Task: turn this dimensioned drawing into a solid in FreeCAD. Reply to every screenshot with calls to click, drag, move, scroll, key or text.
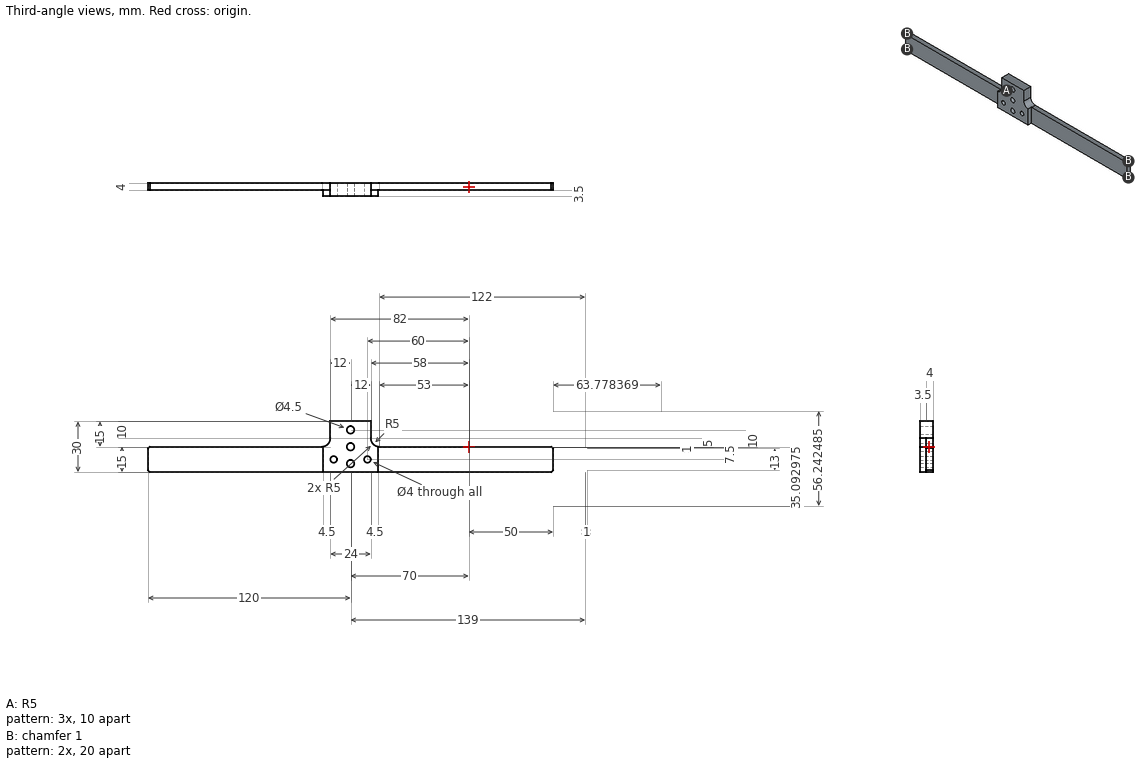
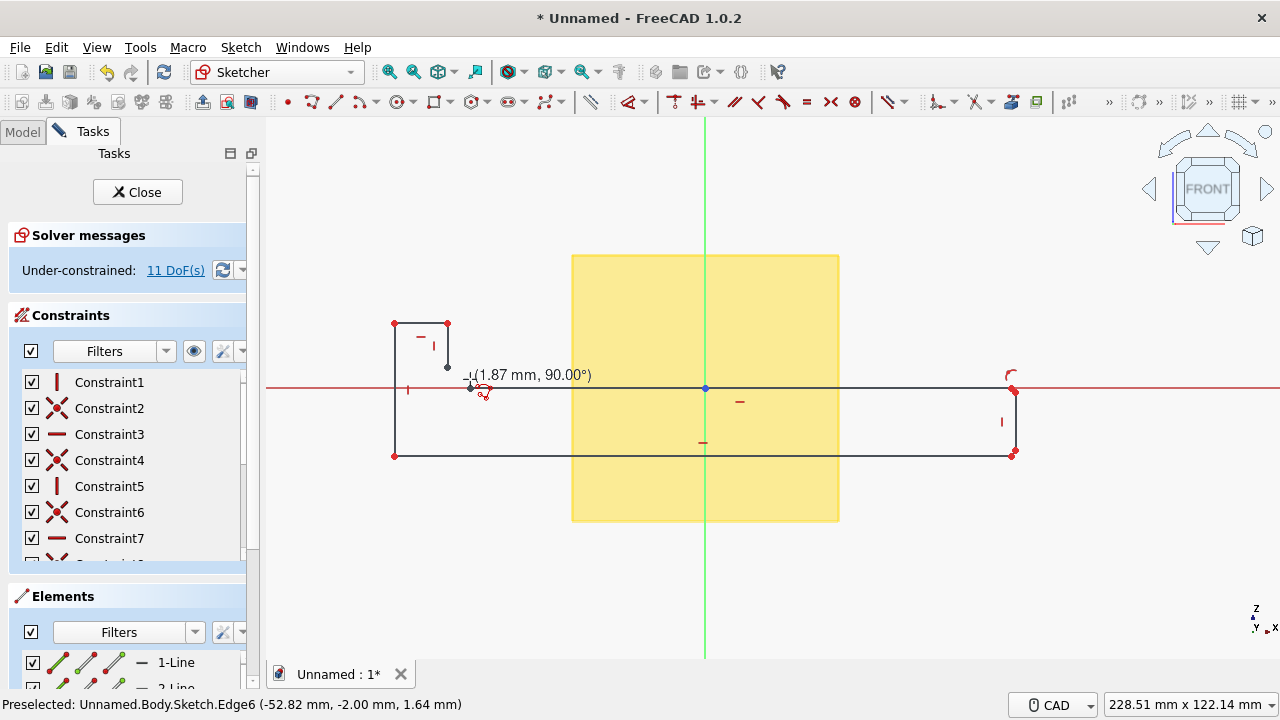
click(378, 102)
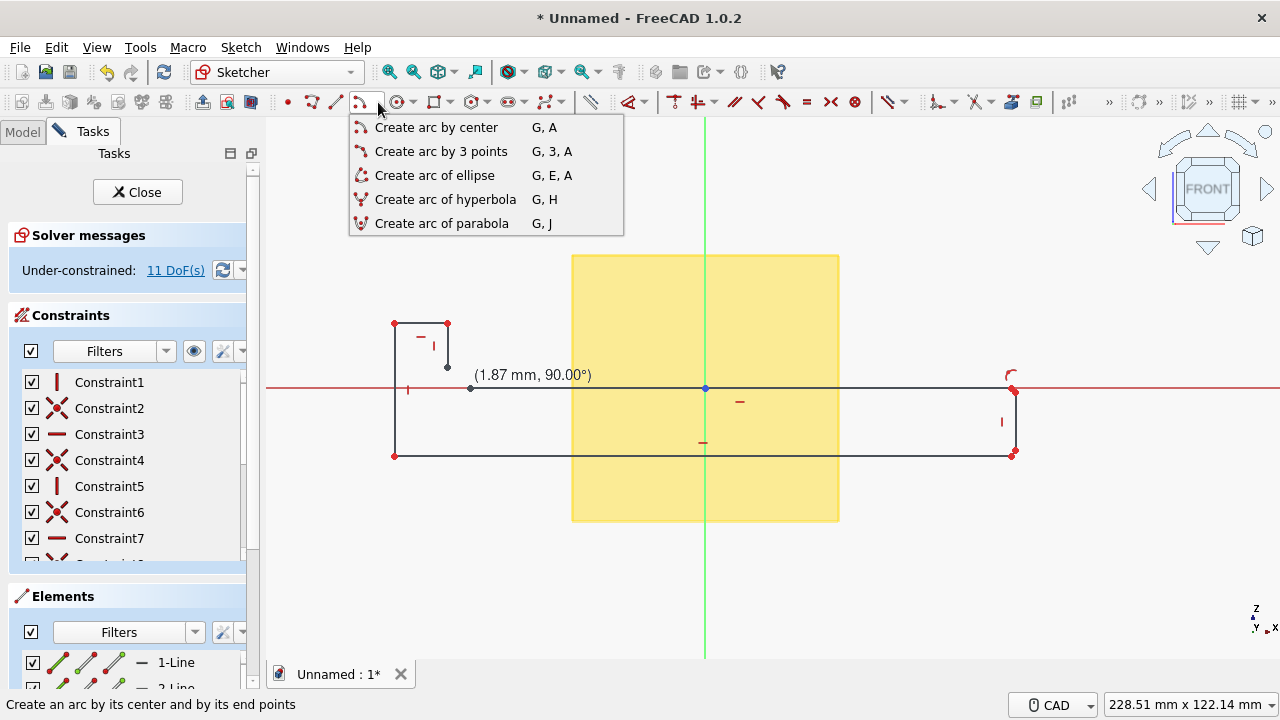
click(486, 151)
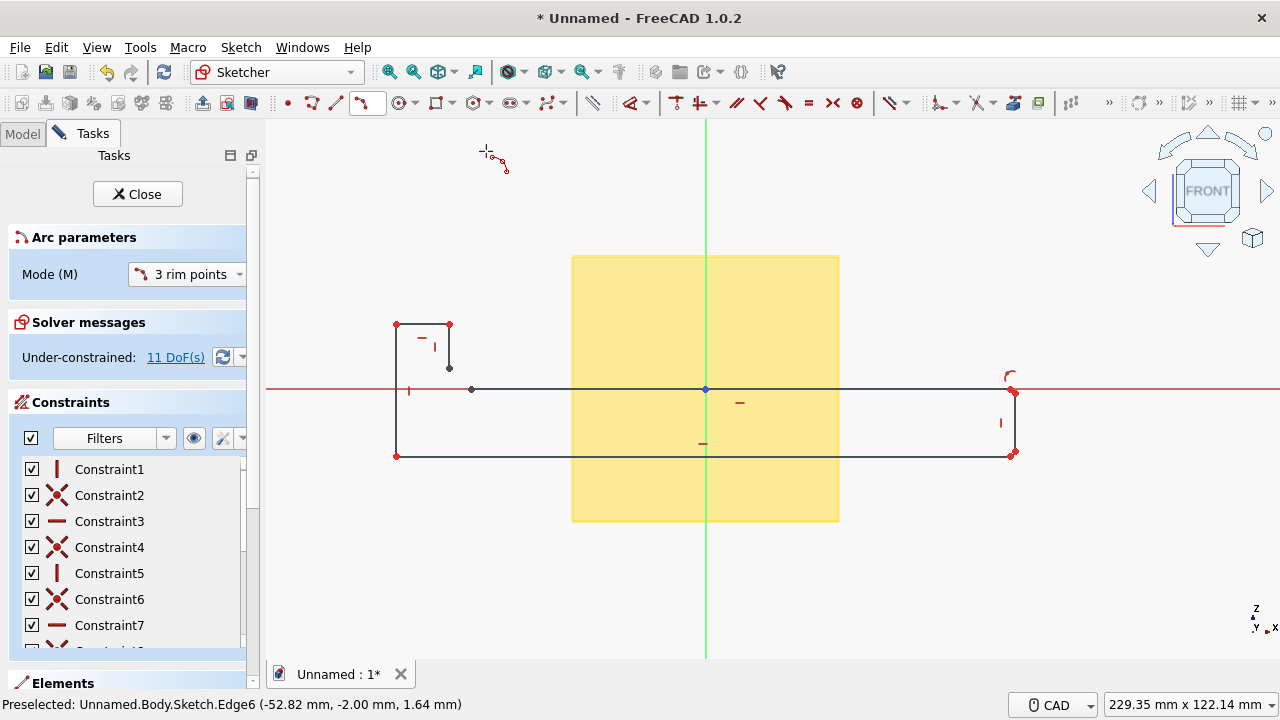
click(471, 380)
click(449, 368)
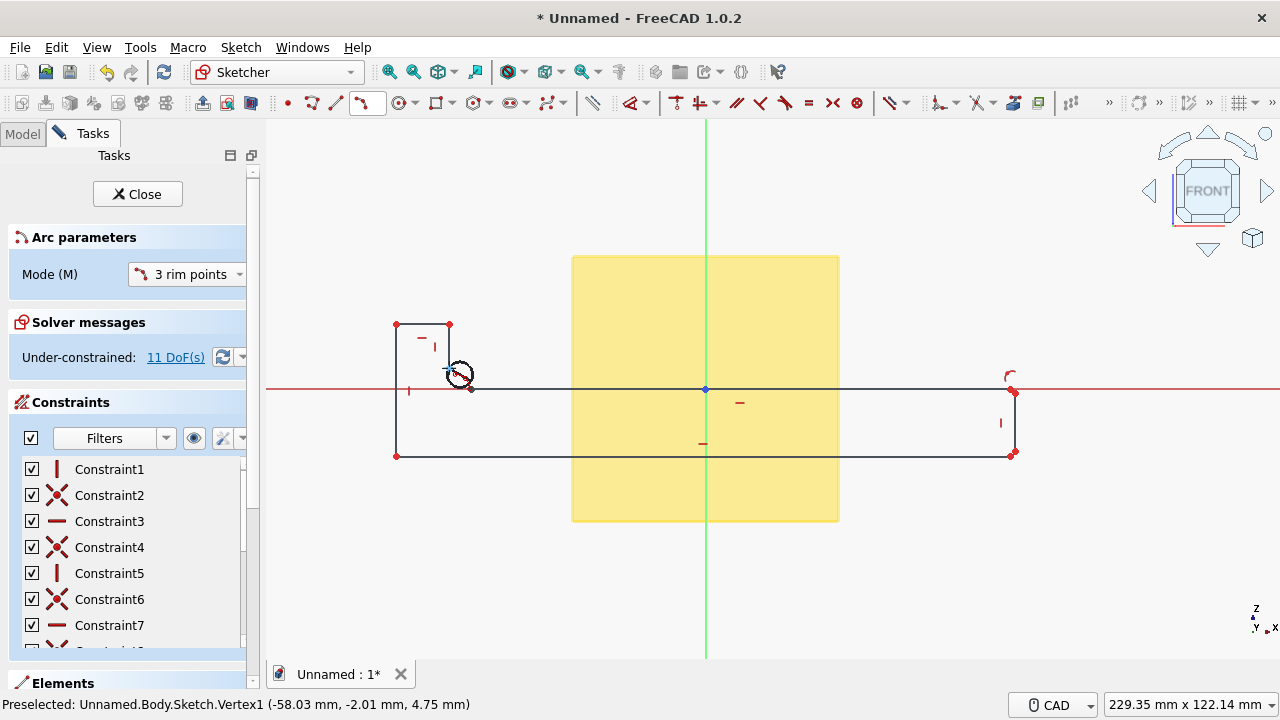
scroll(456, 383, up, 5)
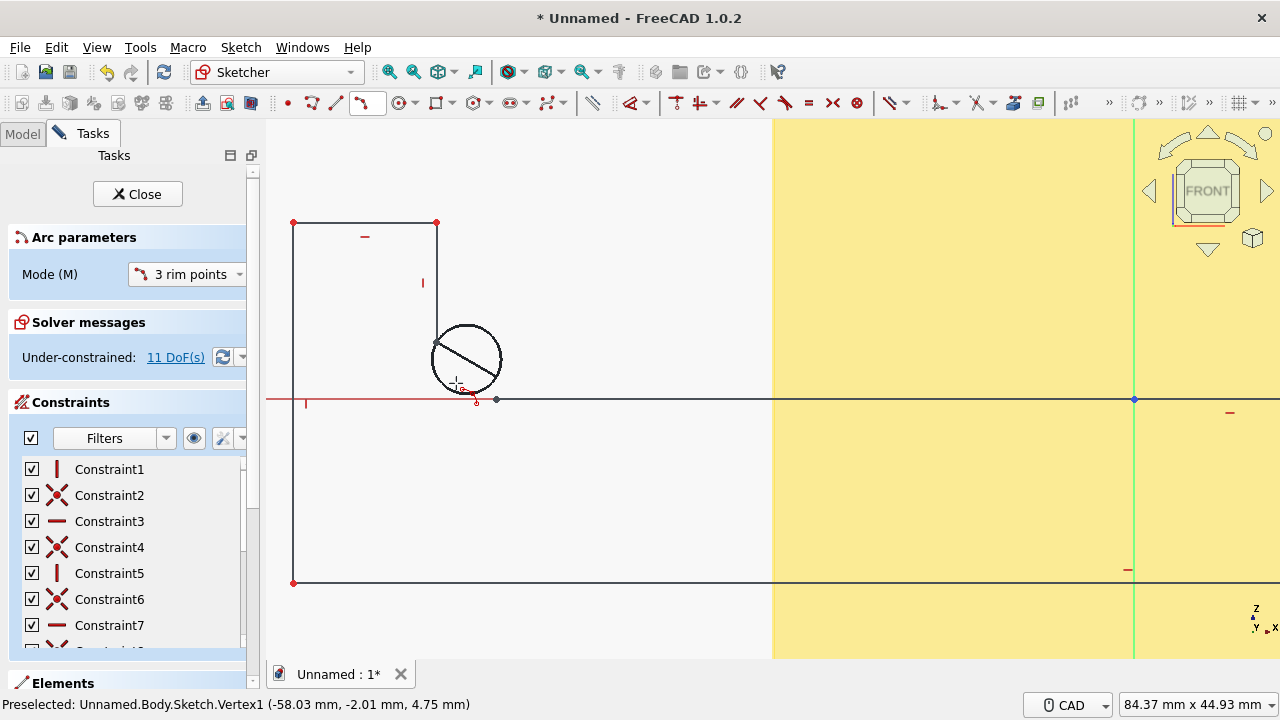
click(455, 382)
key(Escape)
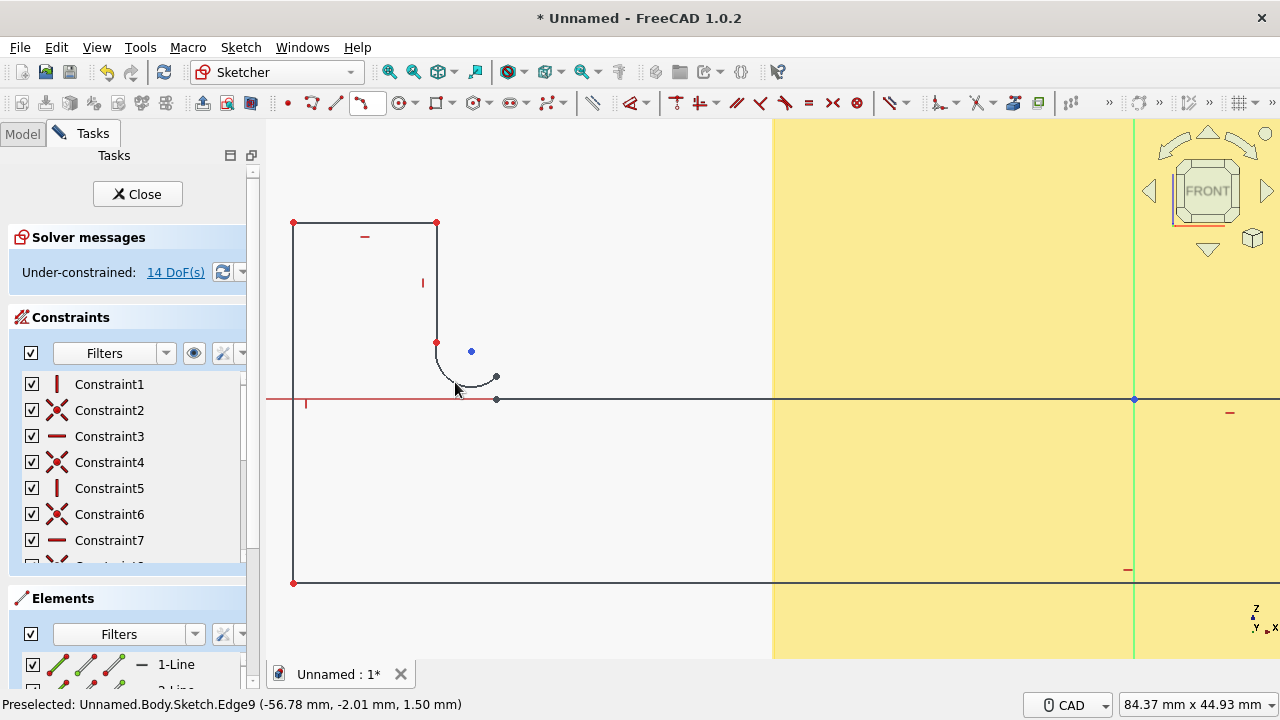
click(437, 306)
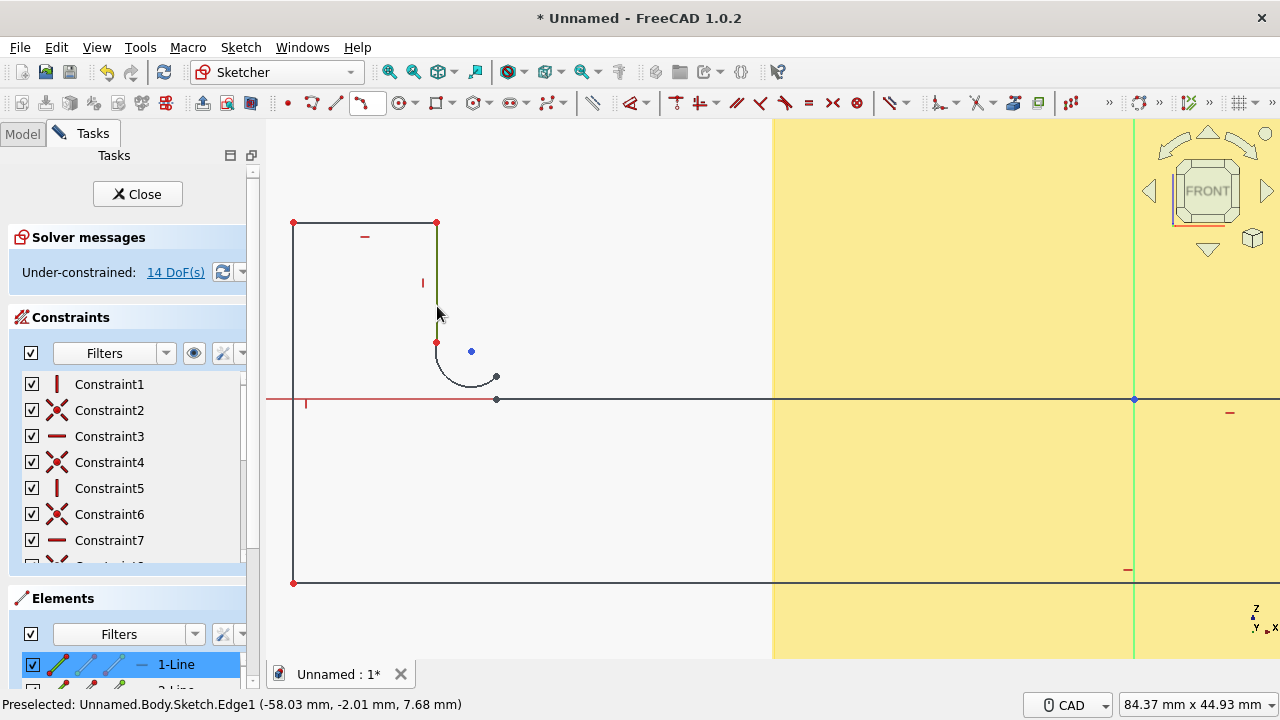
click(440, 369)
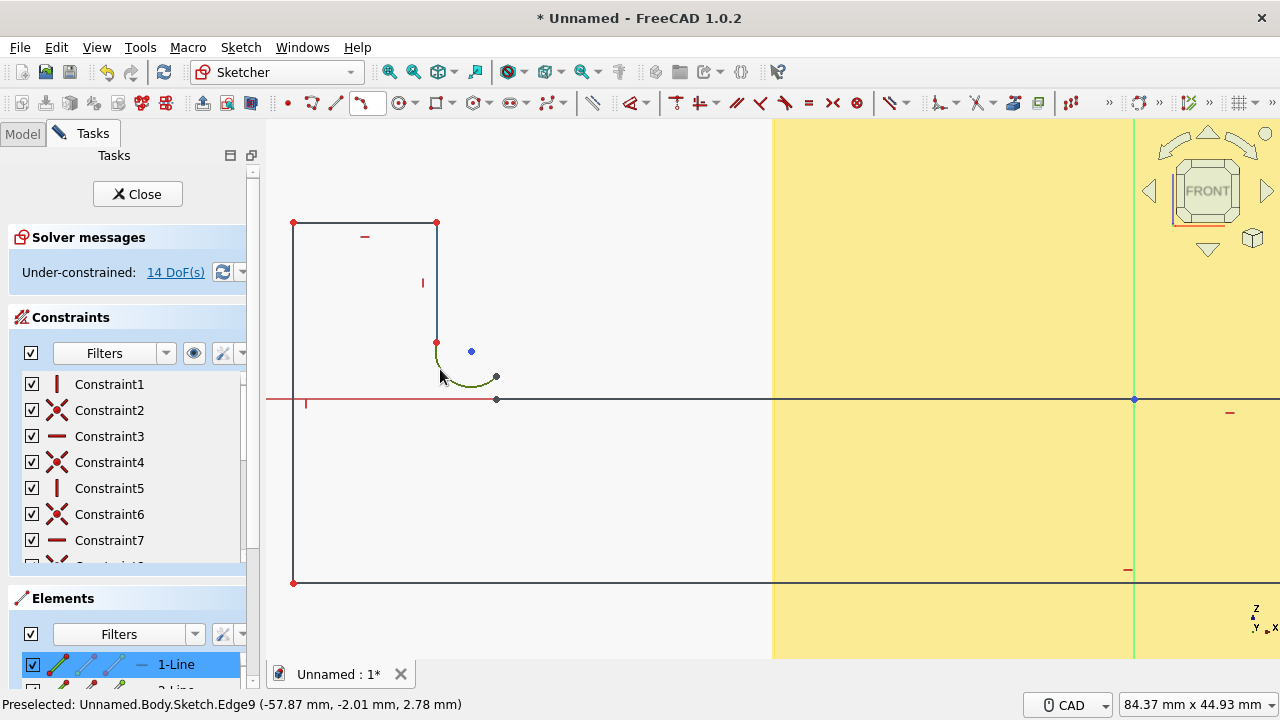
click(786, 104)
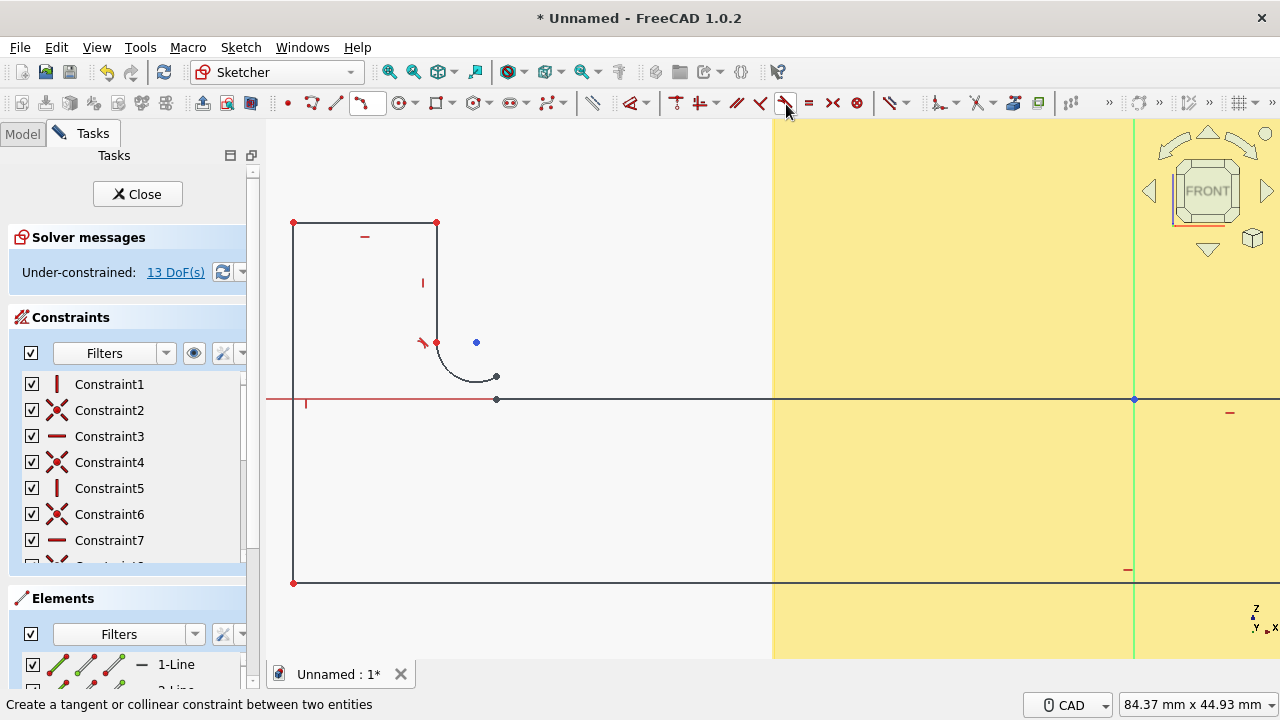
click(937, 399)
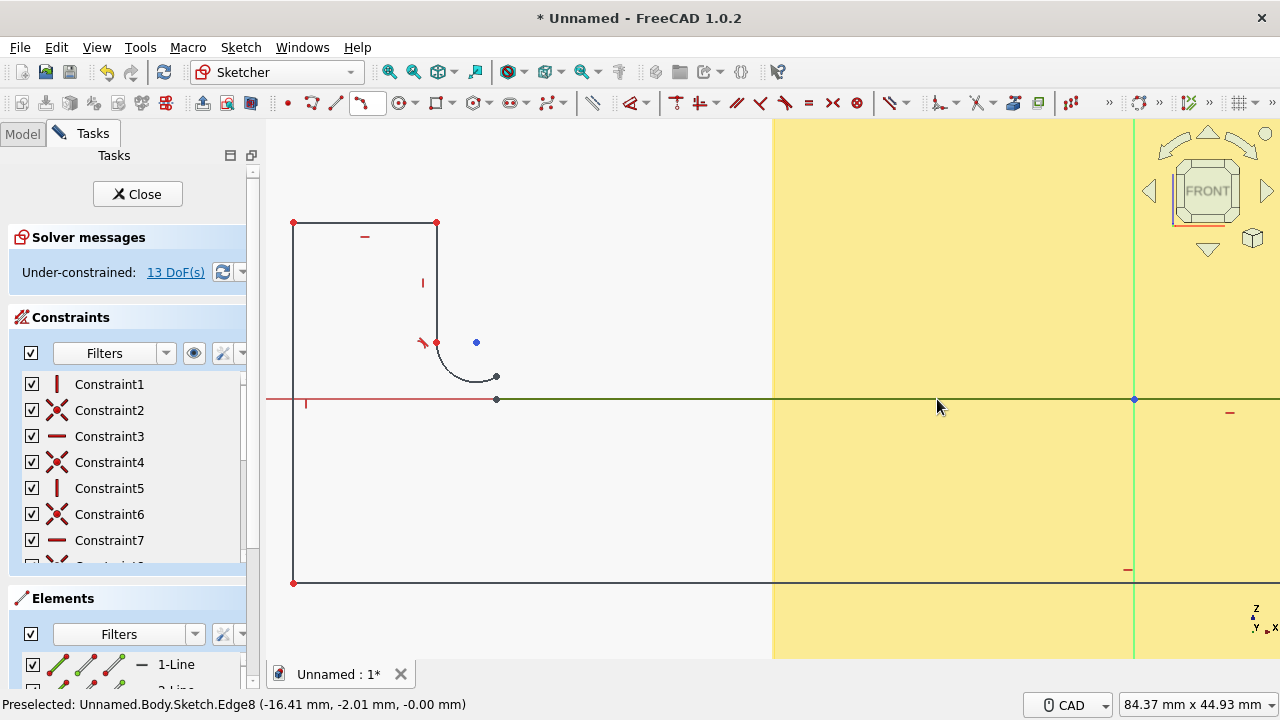
click(444, 366)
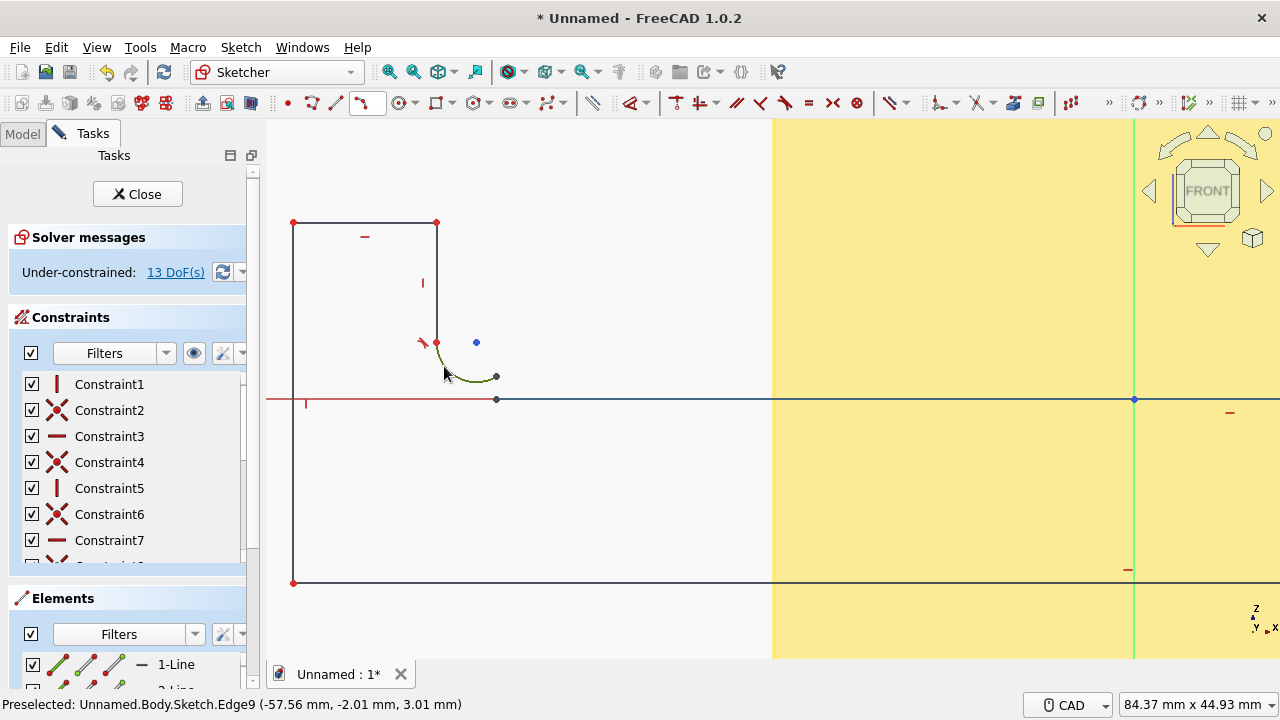
click(786, 104)